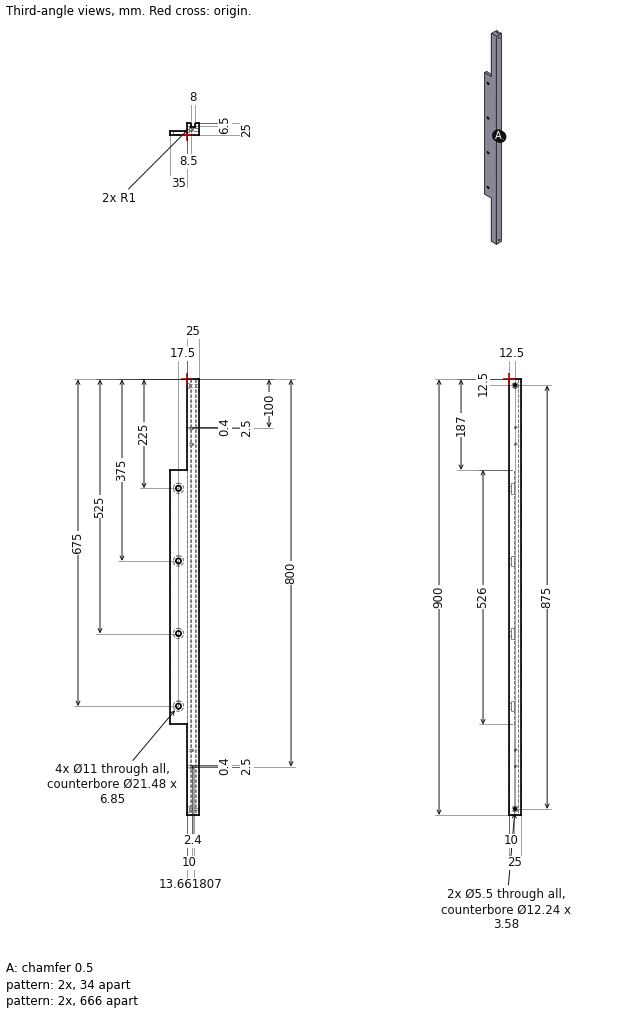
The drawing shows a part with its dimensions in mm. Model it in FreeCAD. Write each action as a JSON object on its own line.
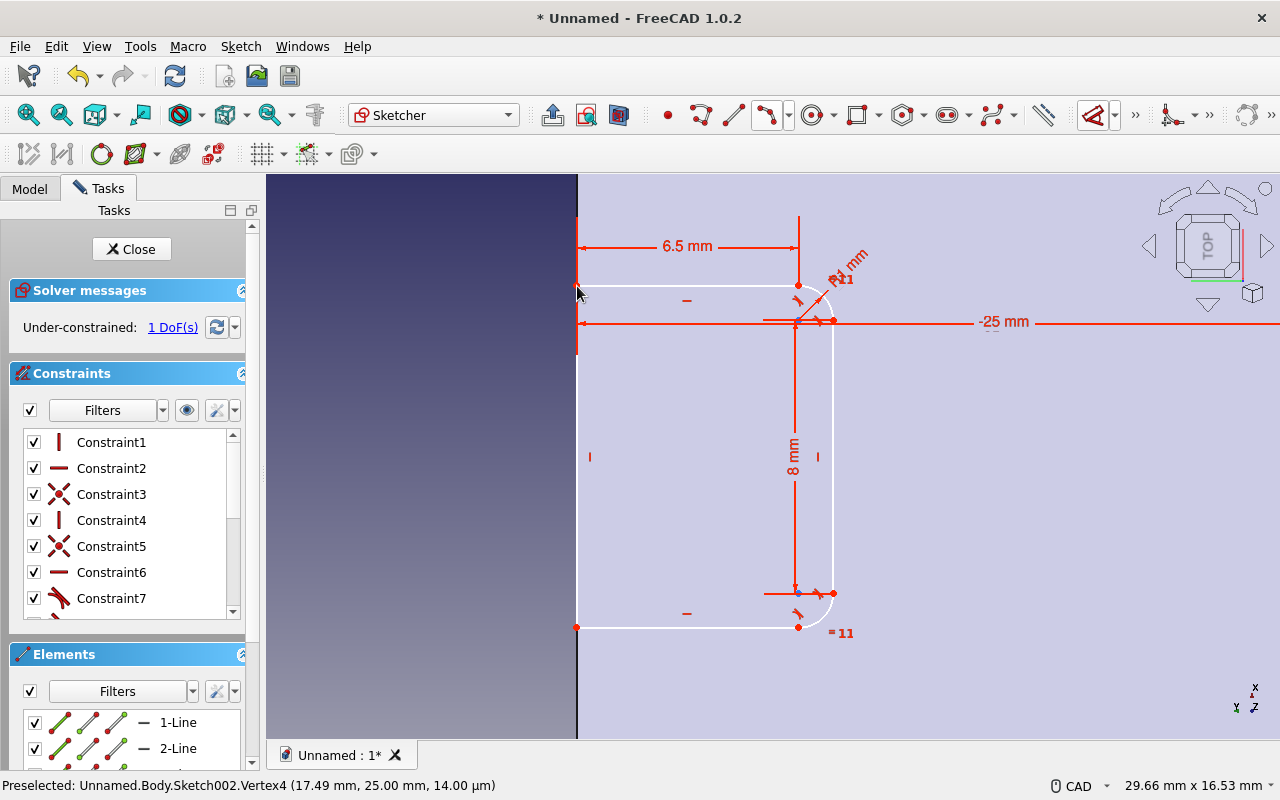
{"action": "left_click", "coordinate": [833, 594]}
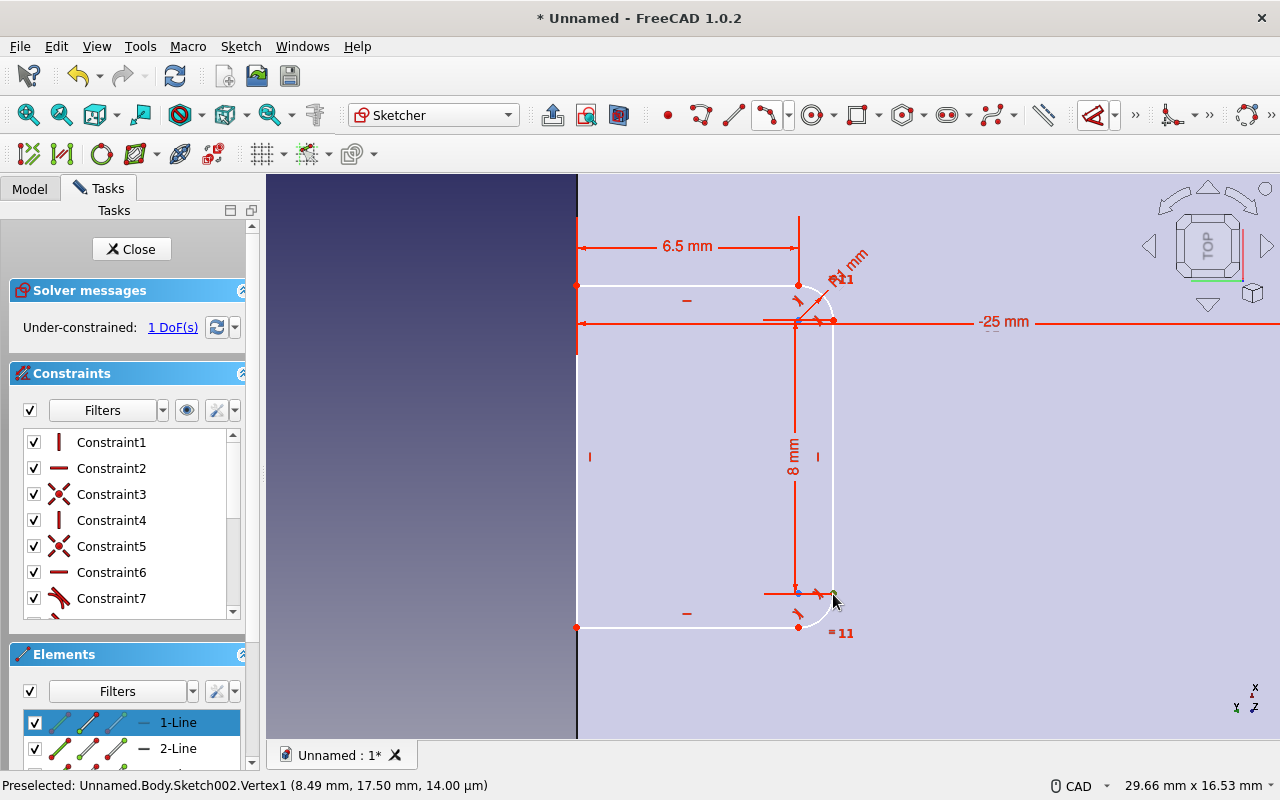
{"action": "key", "text": "i"}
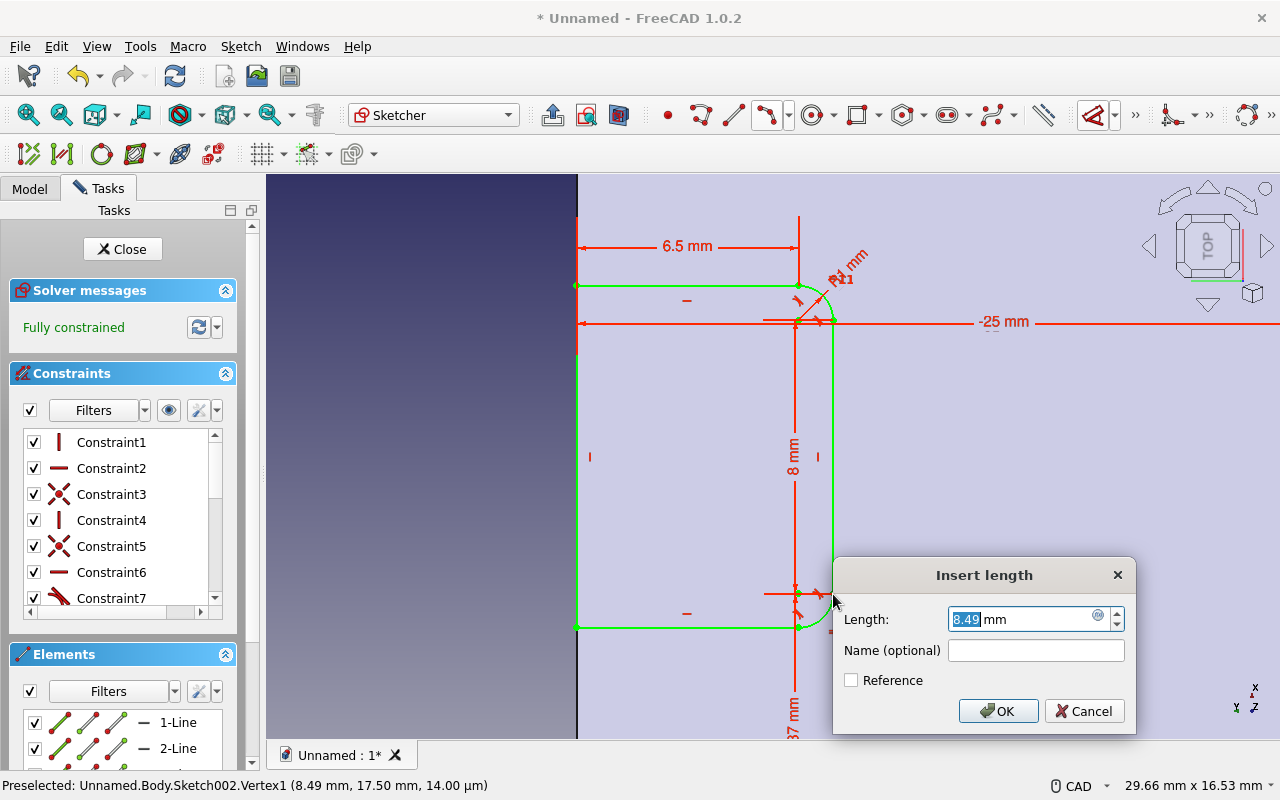
{"action": "type", "text": "8.5"}
{"action": "key", "text": "Return"}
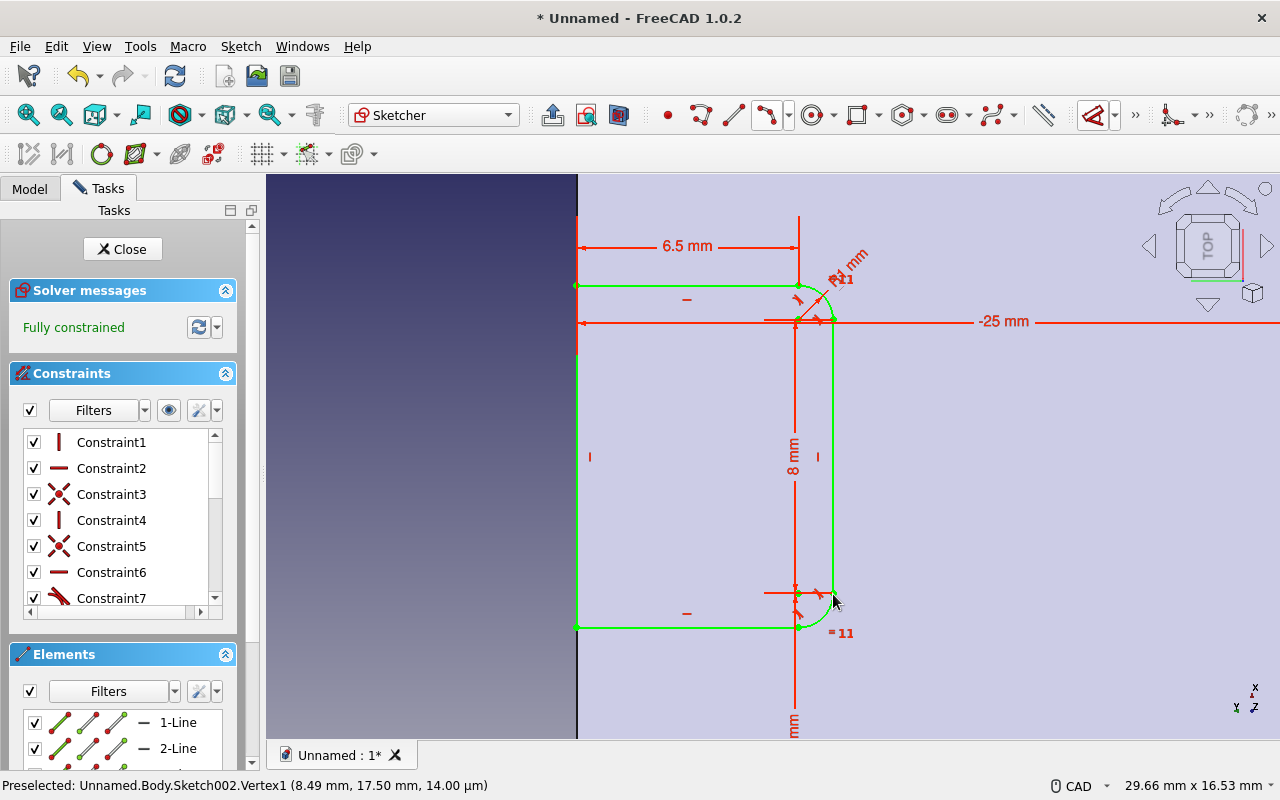
{"action": "left_click", "coordinate": [123, 249]}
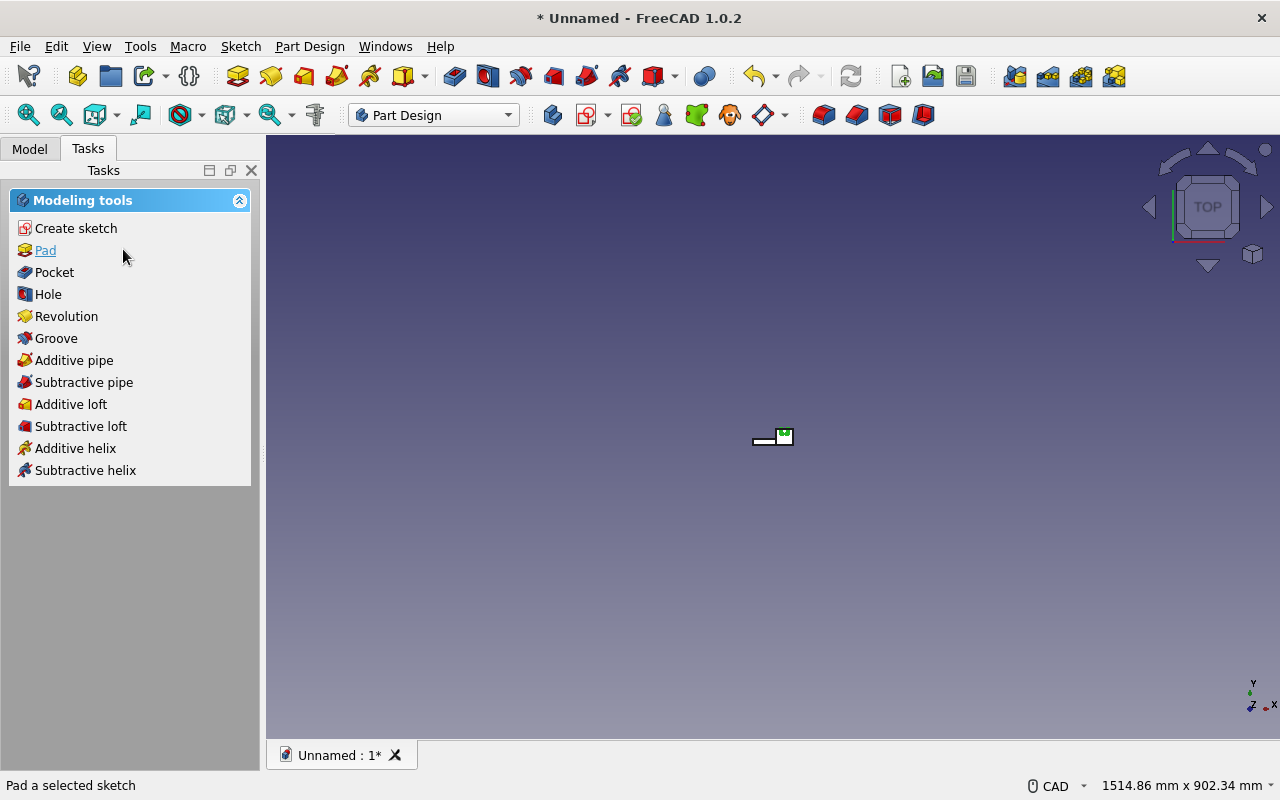
{"action": "left_click", "coordinate": [455, 76]}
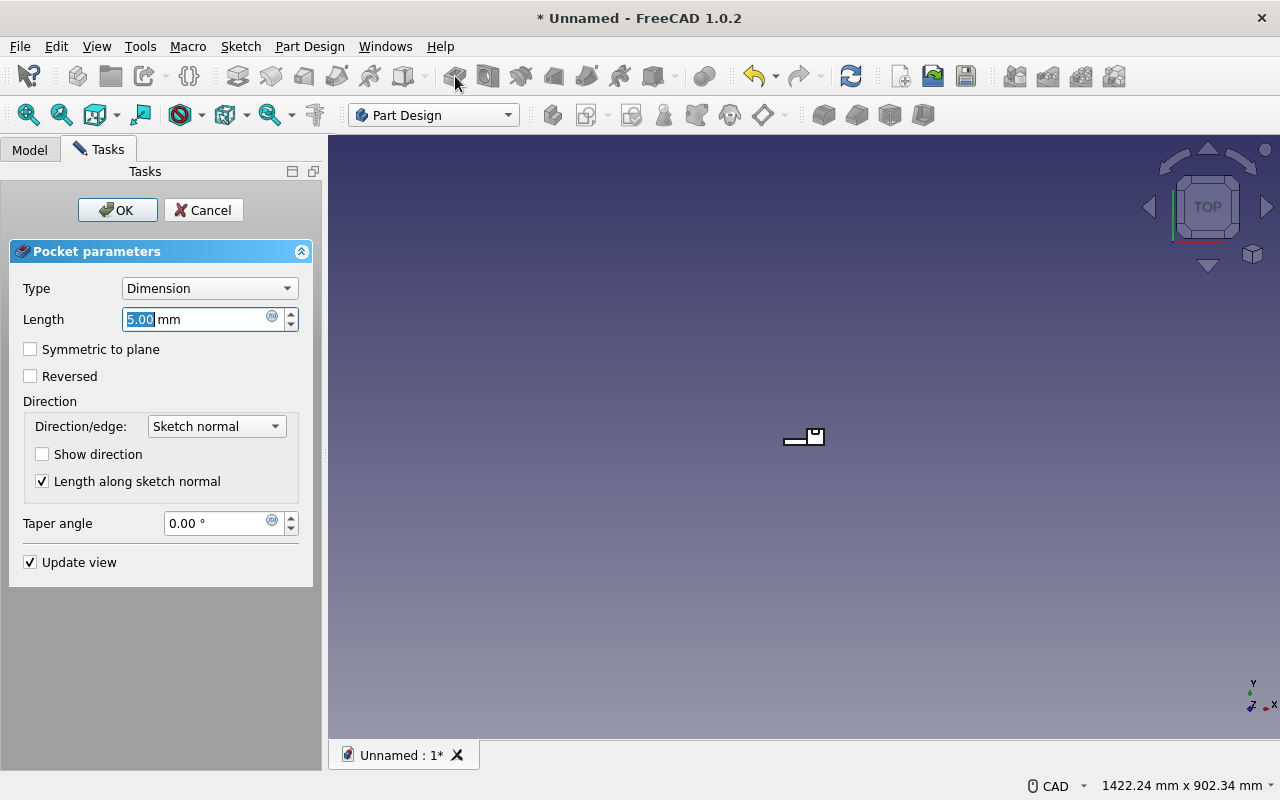
{"action": "left_click", "coordinate": [210, 288]}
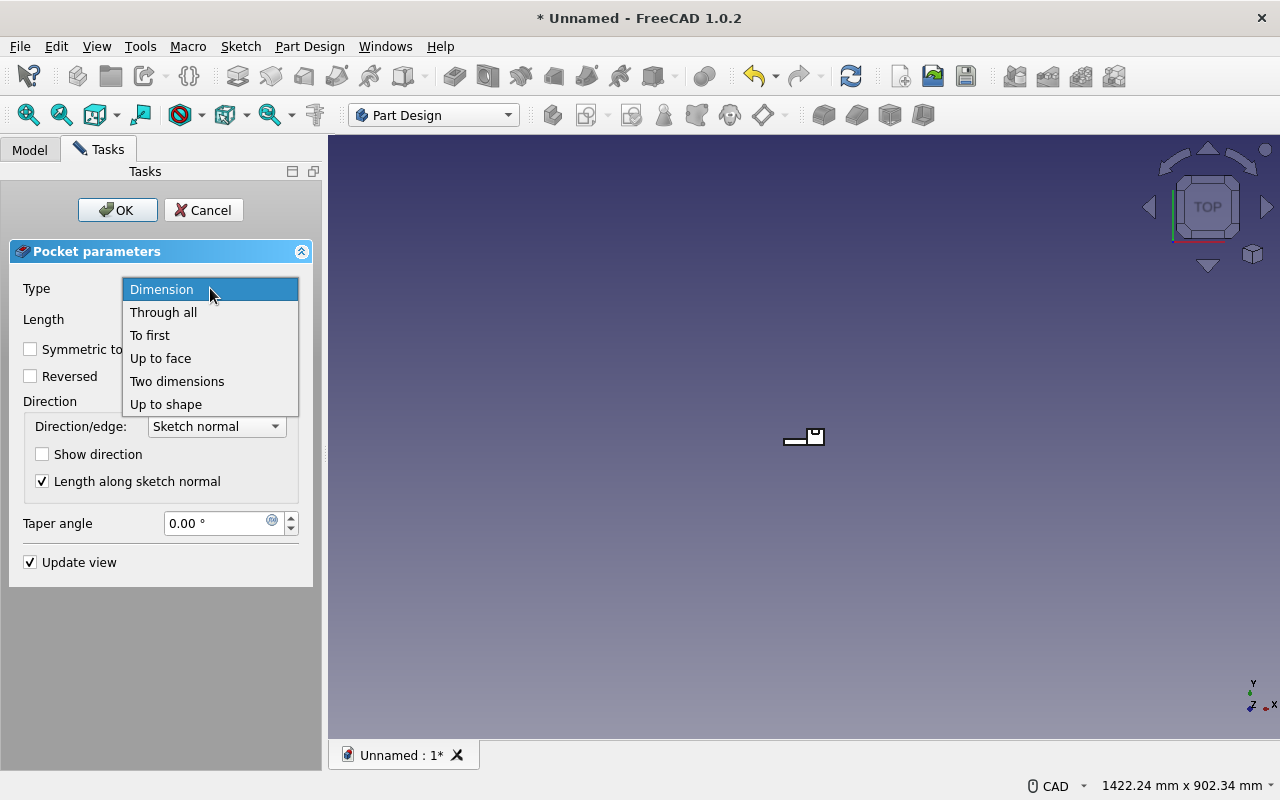
{"action": "left_click", "coordinate": [208, 312]}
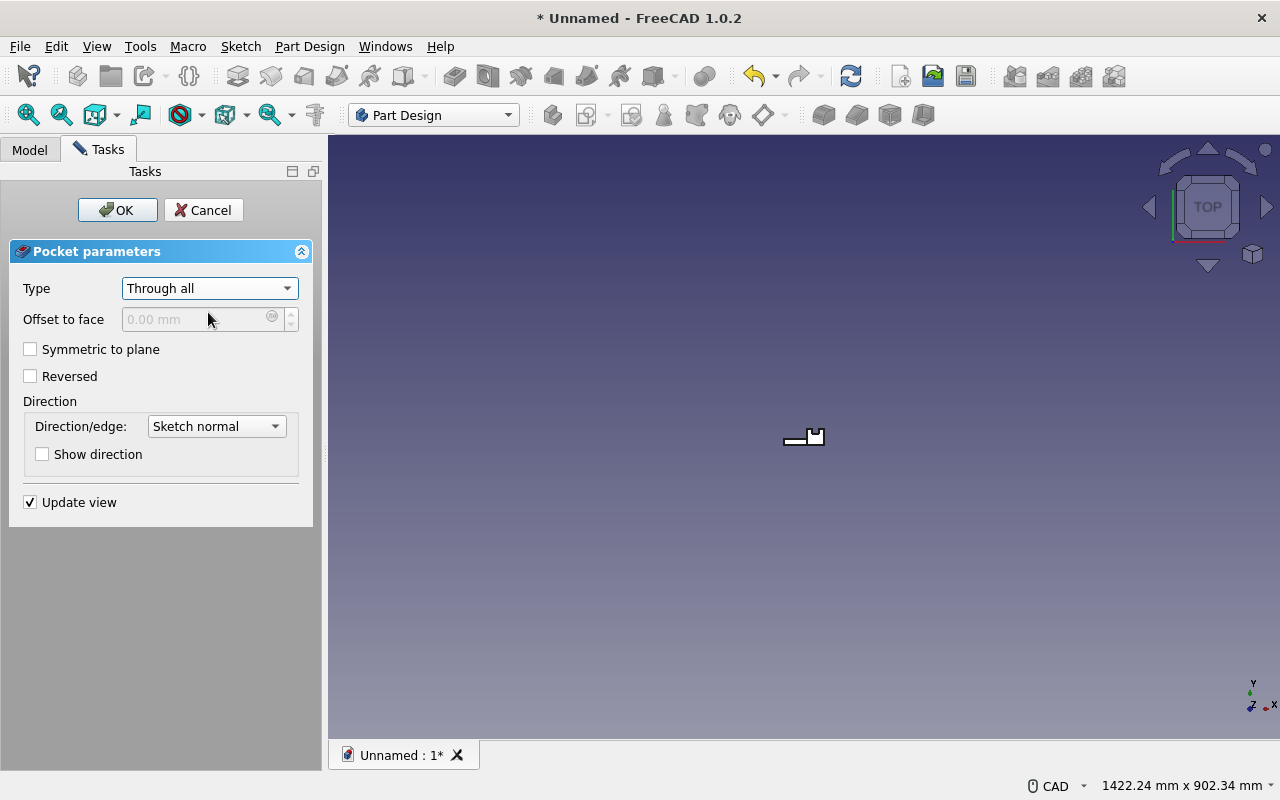
{"action": "left_click", "coordinate": [118, 210]}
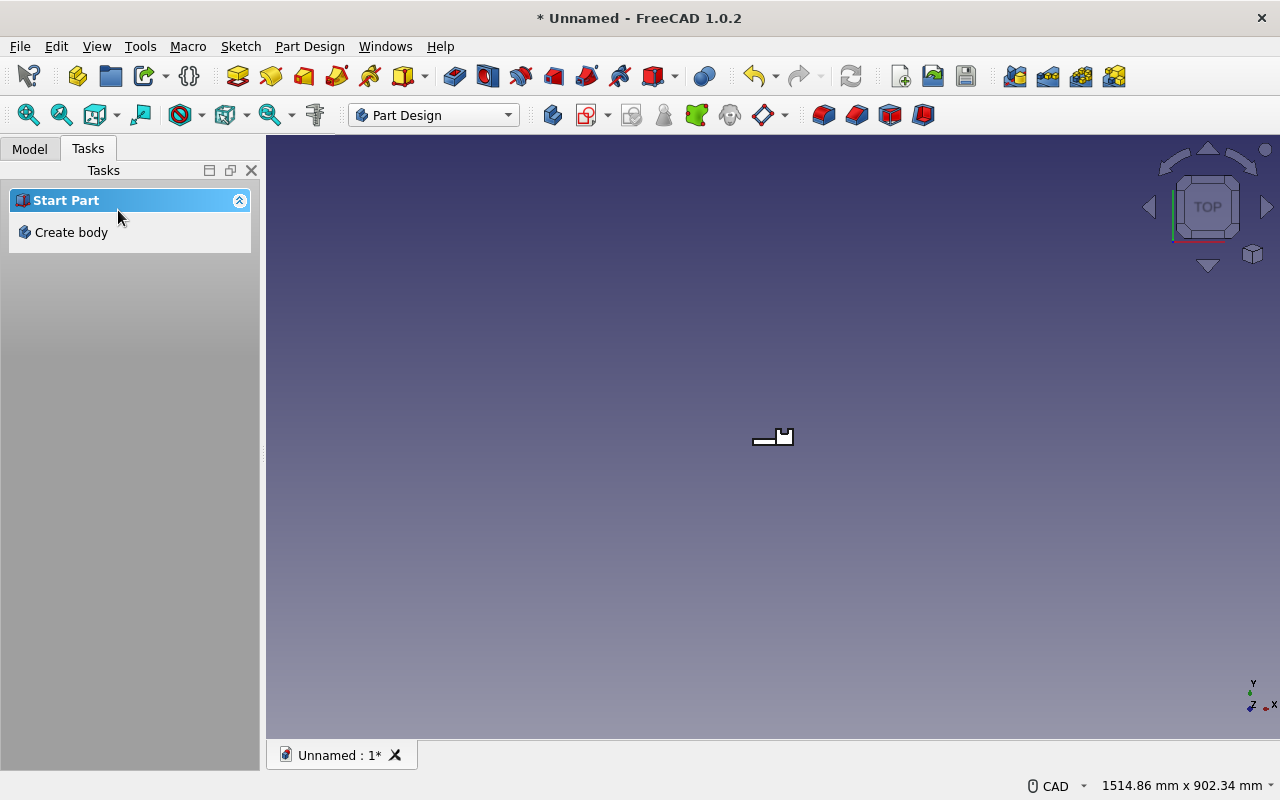
{"action": "left_click", "coordinate": [29, 116]}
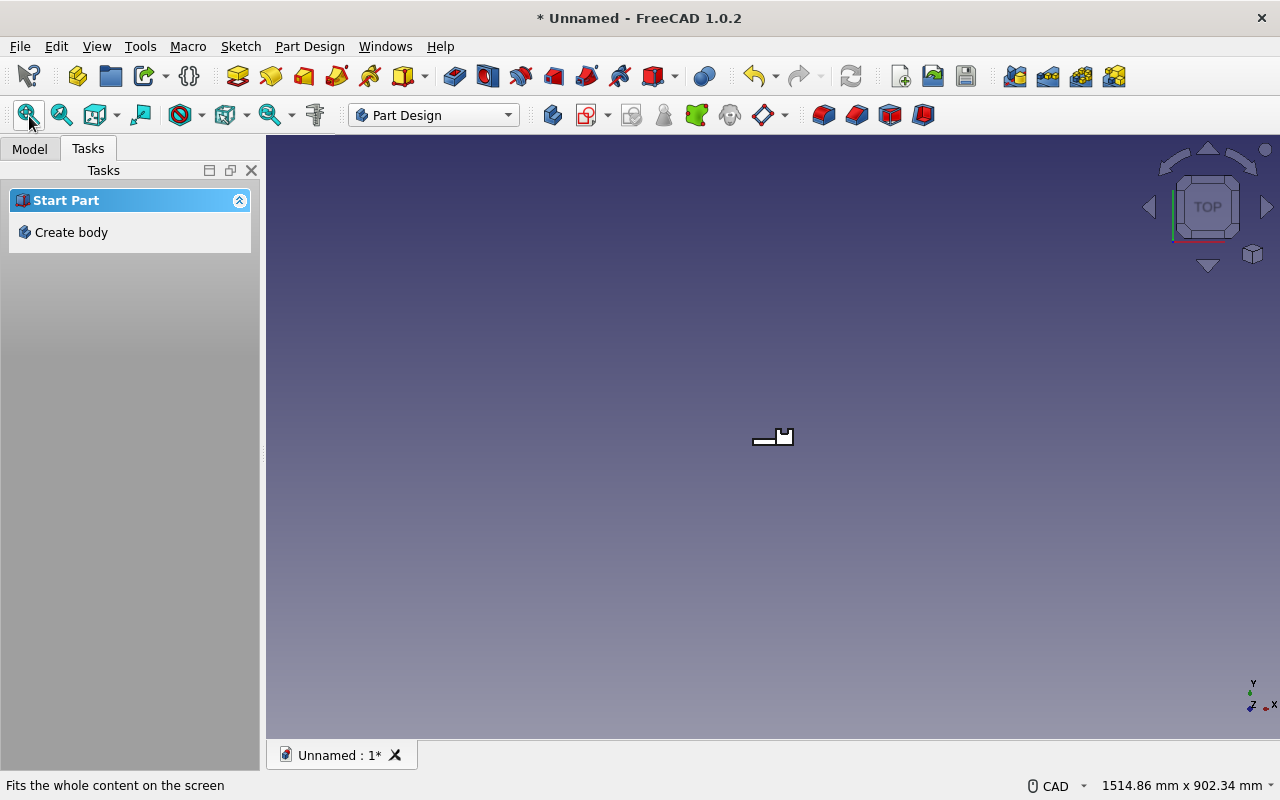
{"action": "key", "text": "0"}